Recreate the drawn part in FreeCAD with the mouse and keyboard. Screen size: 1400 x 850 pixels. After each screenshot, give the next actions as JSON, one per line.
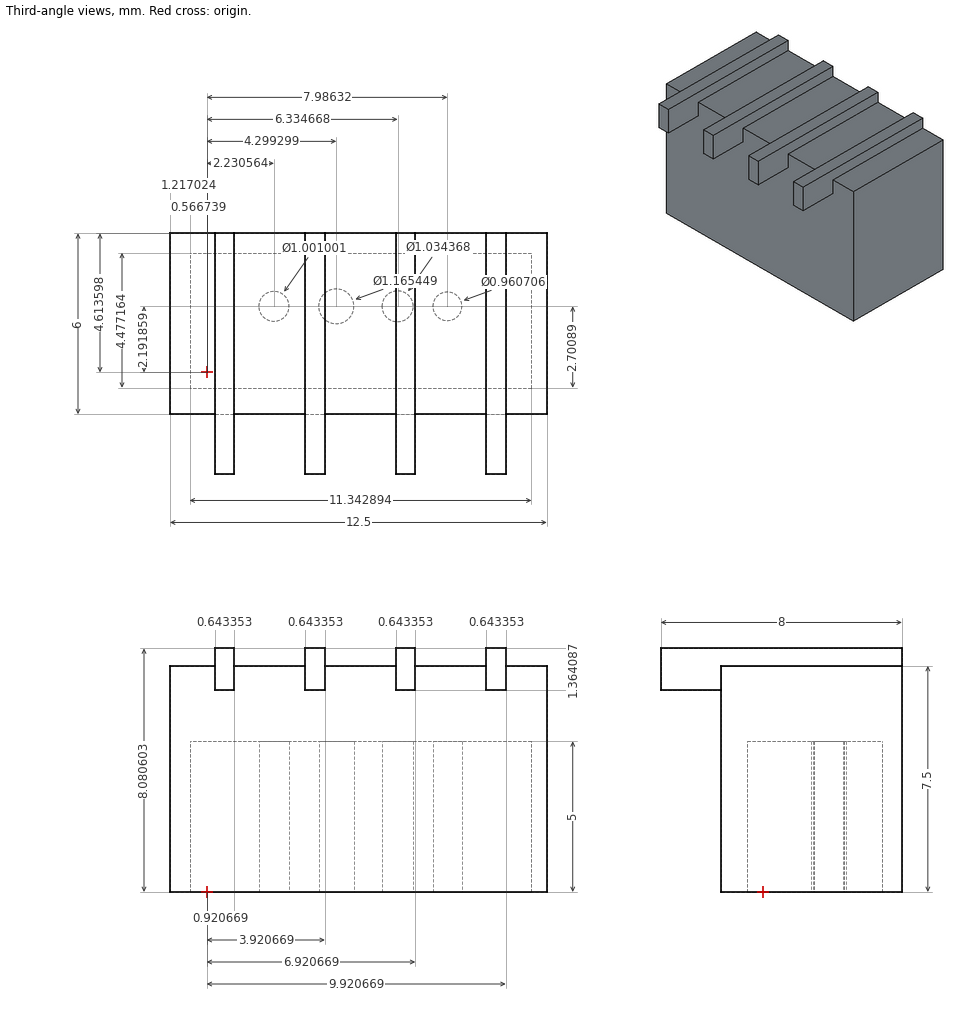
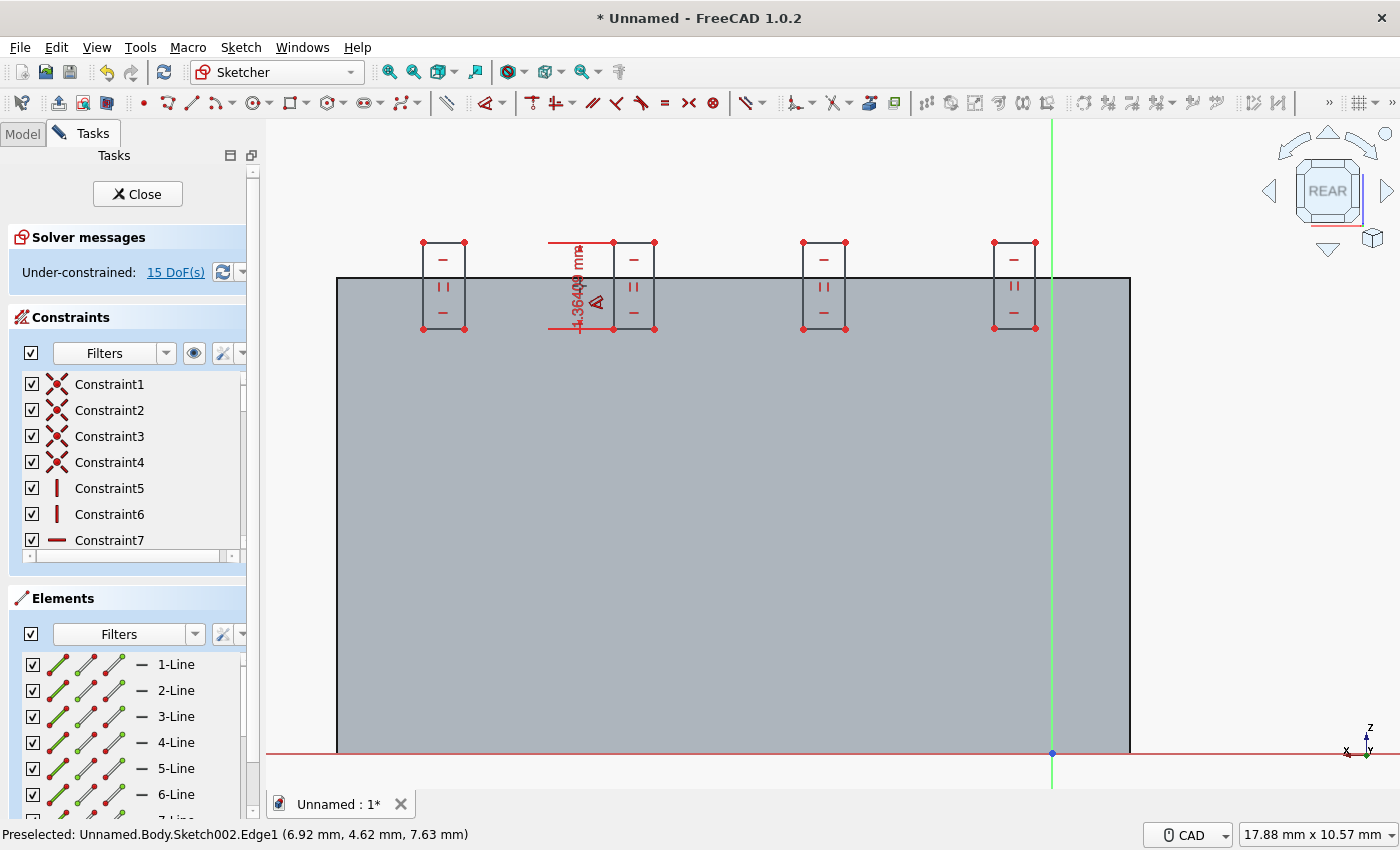
{"action": "left_click", "coordinate": [626, 329]}
{"action": "left_click", "coordinate": [634, 363]}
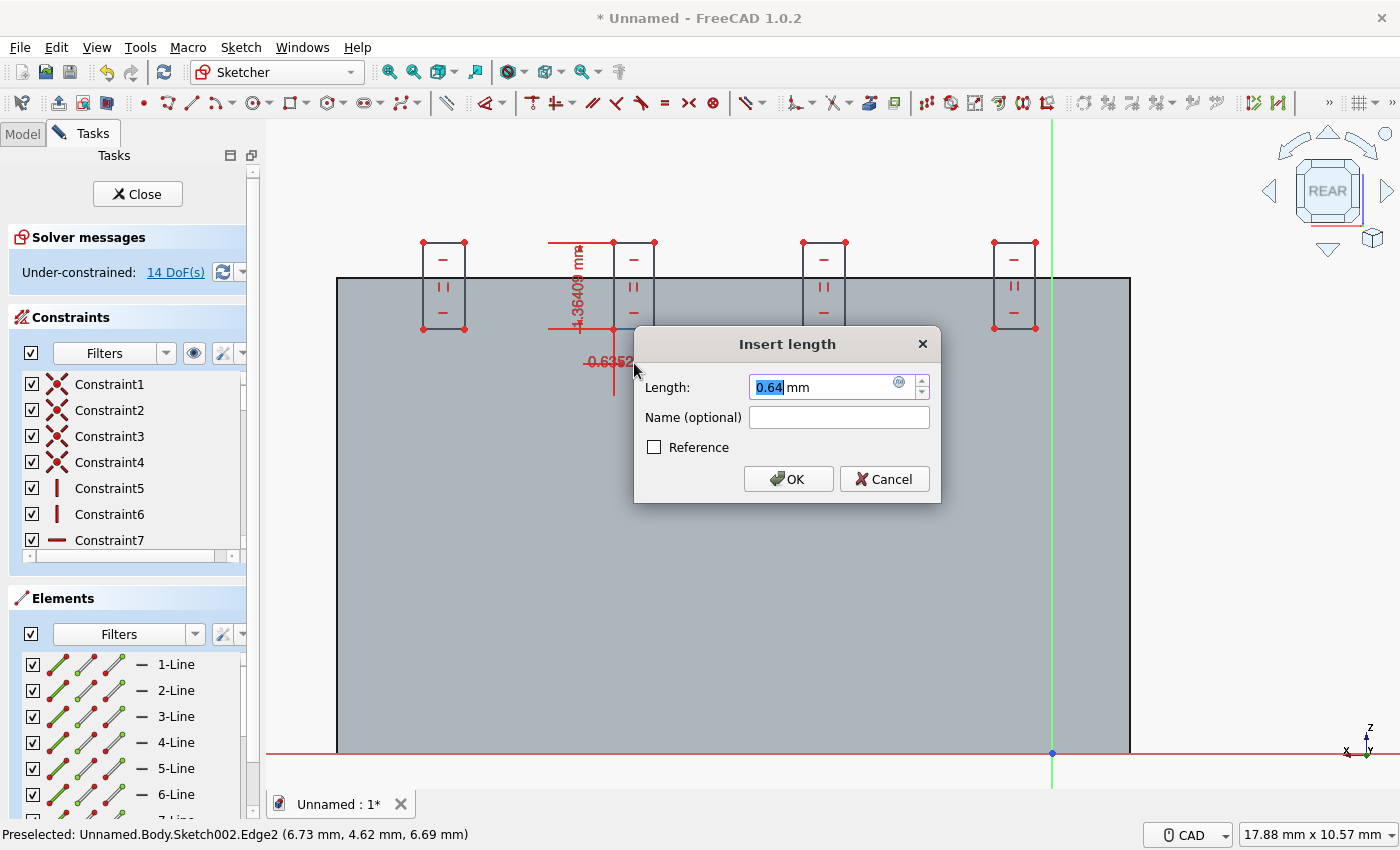
{"action": "type", "text": "0.643353"}
{"action": "key", "text": "Return"}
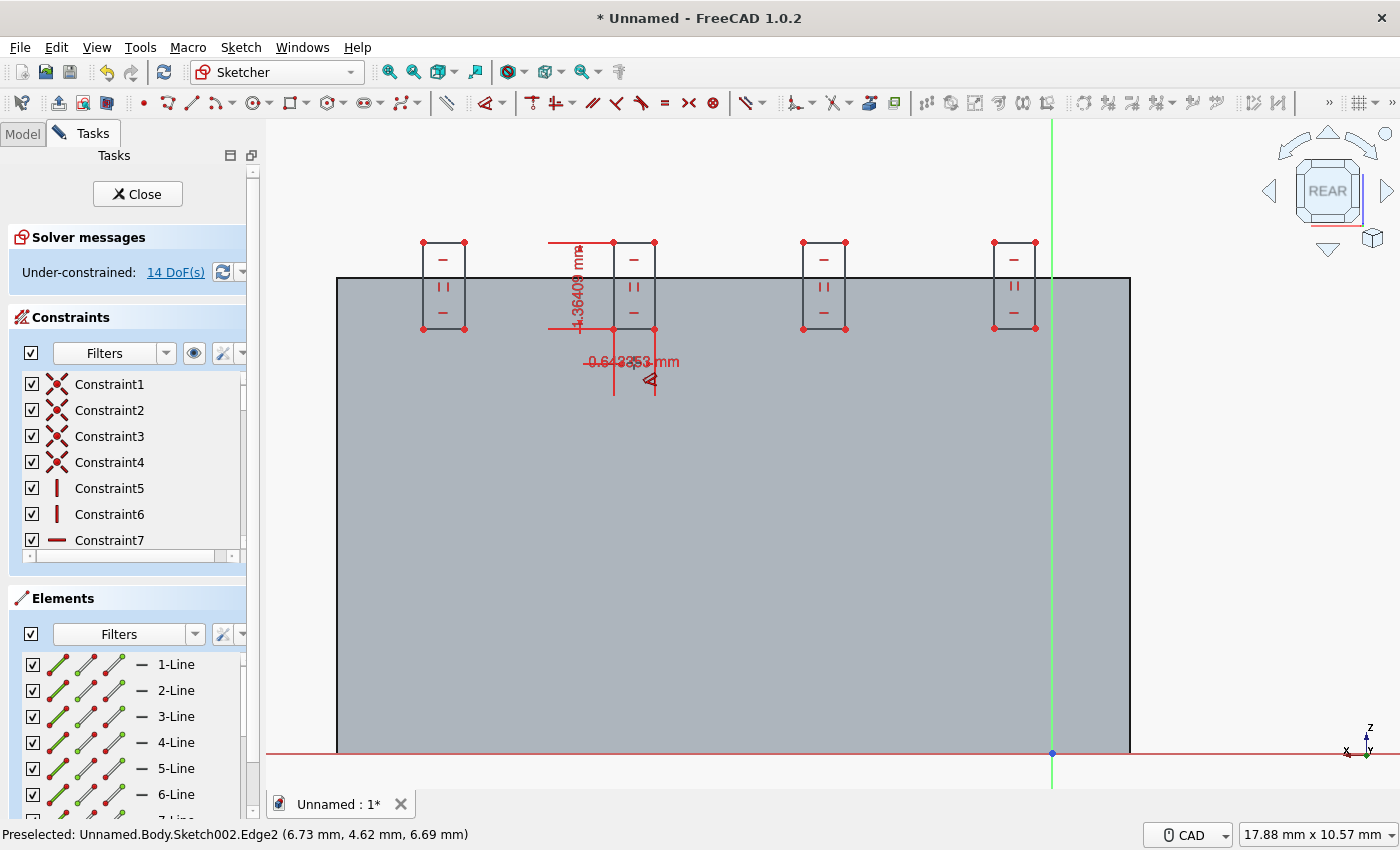
{"action": "left_click", "coordinate": [423, 269]}
{"action": "left_click", "coordinate": [389, 286]}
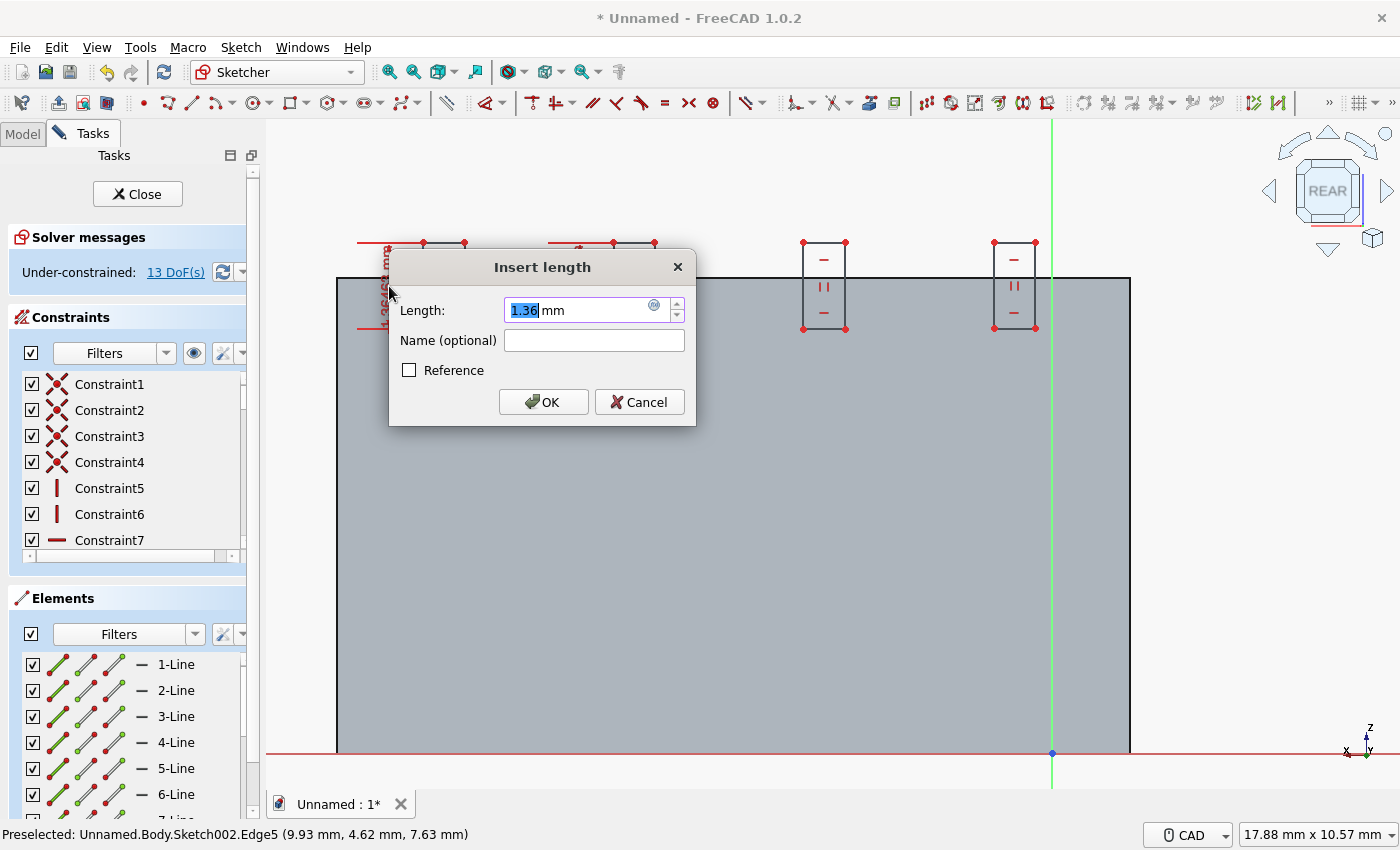
{"action": "type", "text": "1.364087"}
{"action": "key", "text": "Return"}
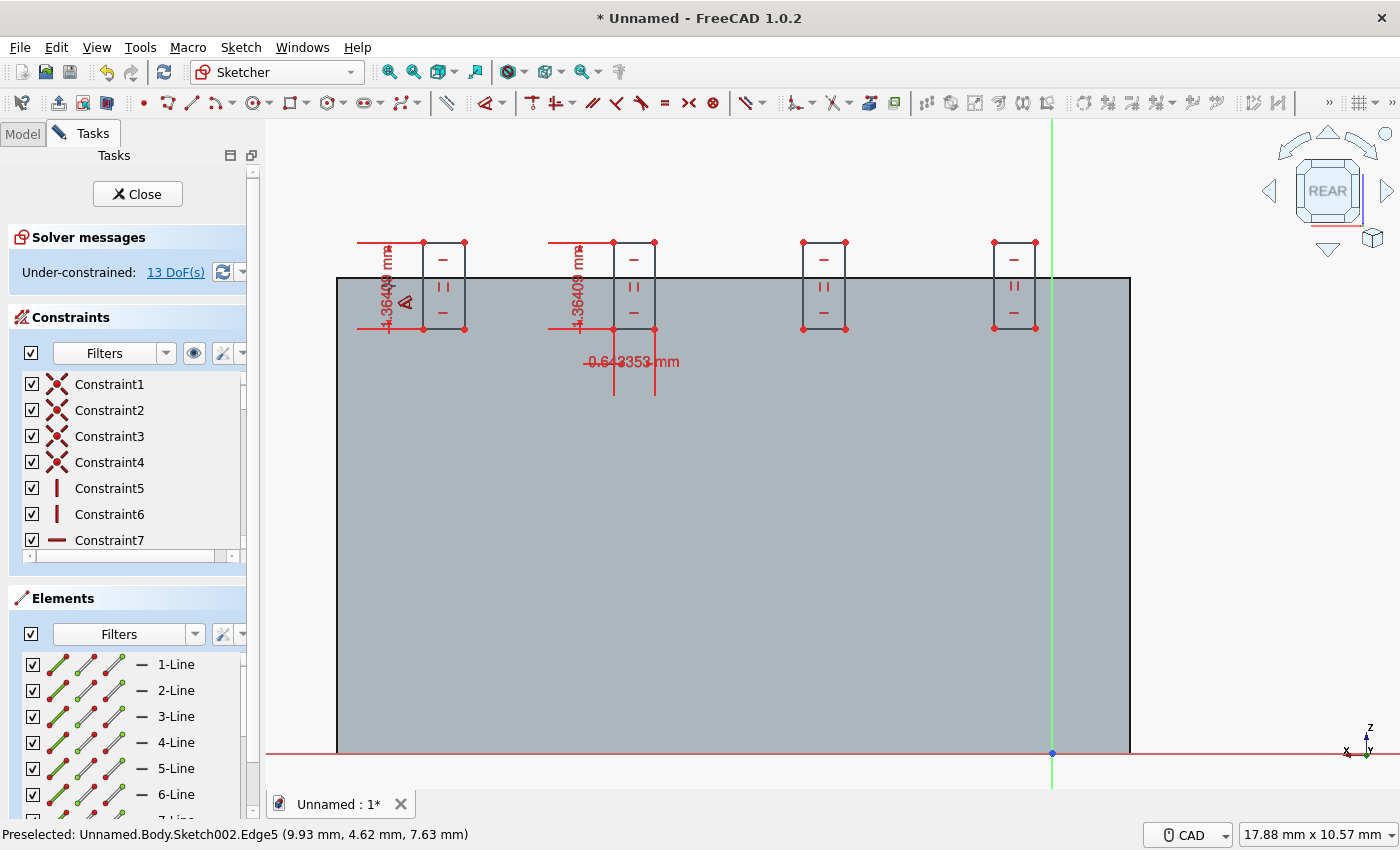
{"action": "left_click", "coordinate": [436, 329]}
{"action": "left_click", "coordinate": [444, 363]}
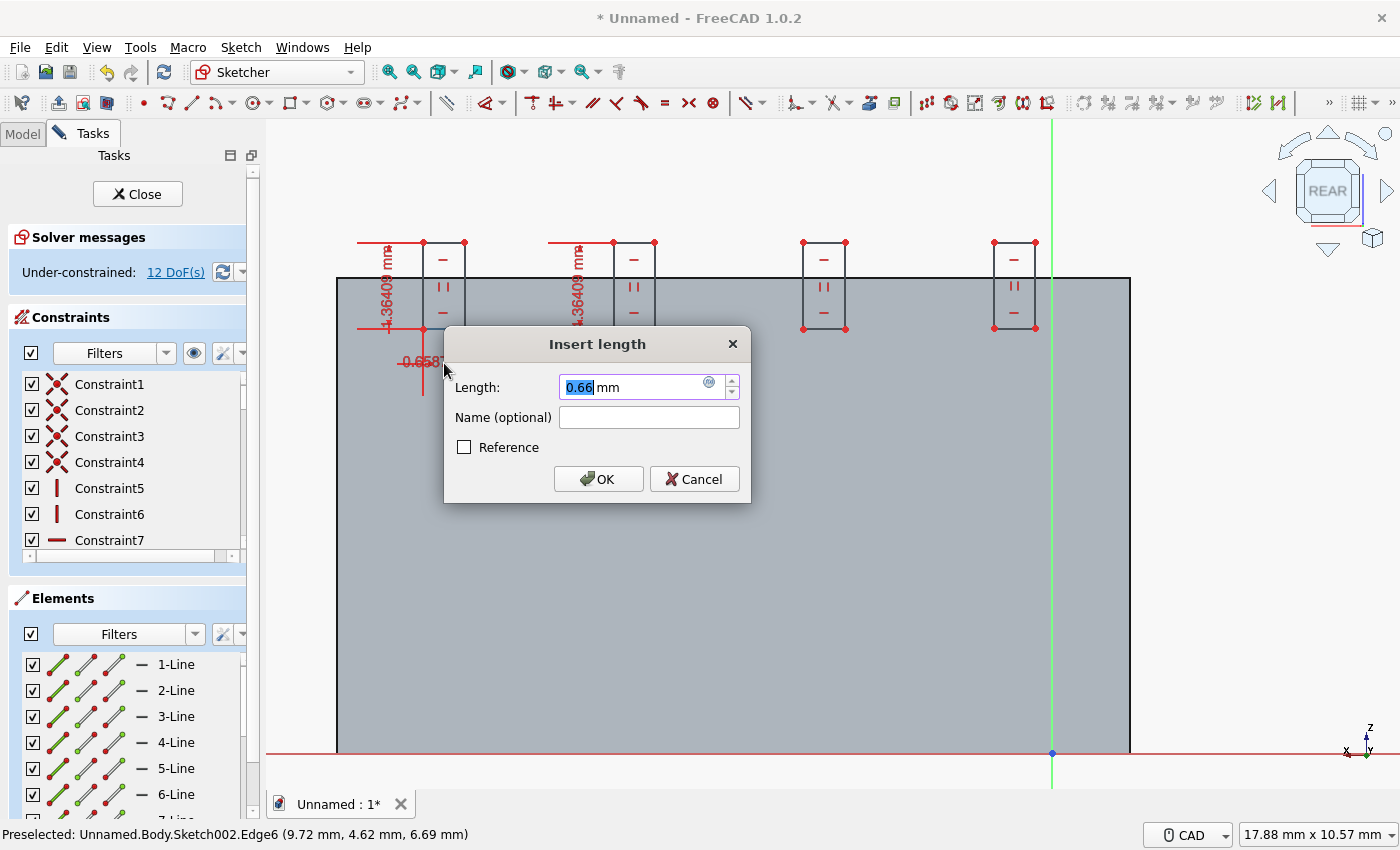
{"action": "type", "text": "0.643353"}
{"action": "key", "text": "Return"}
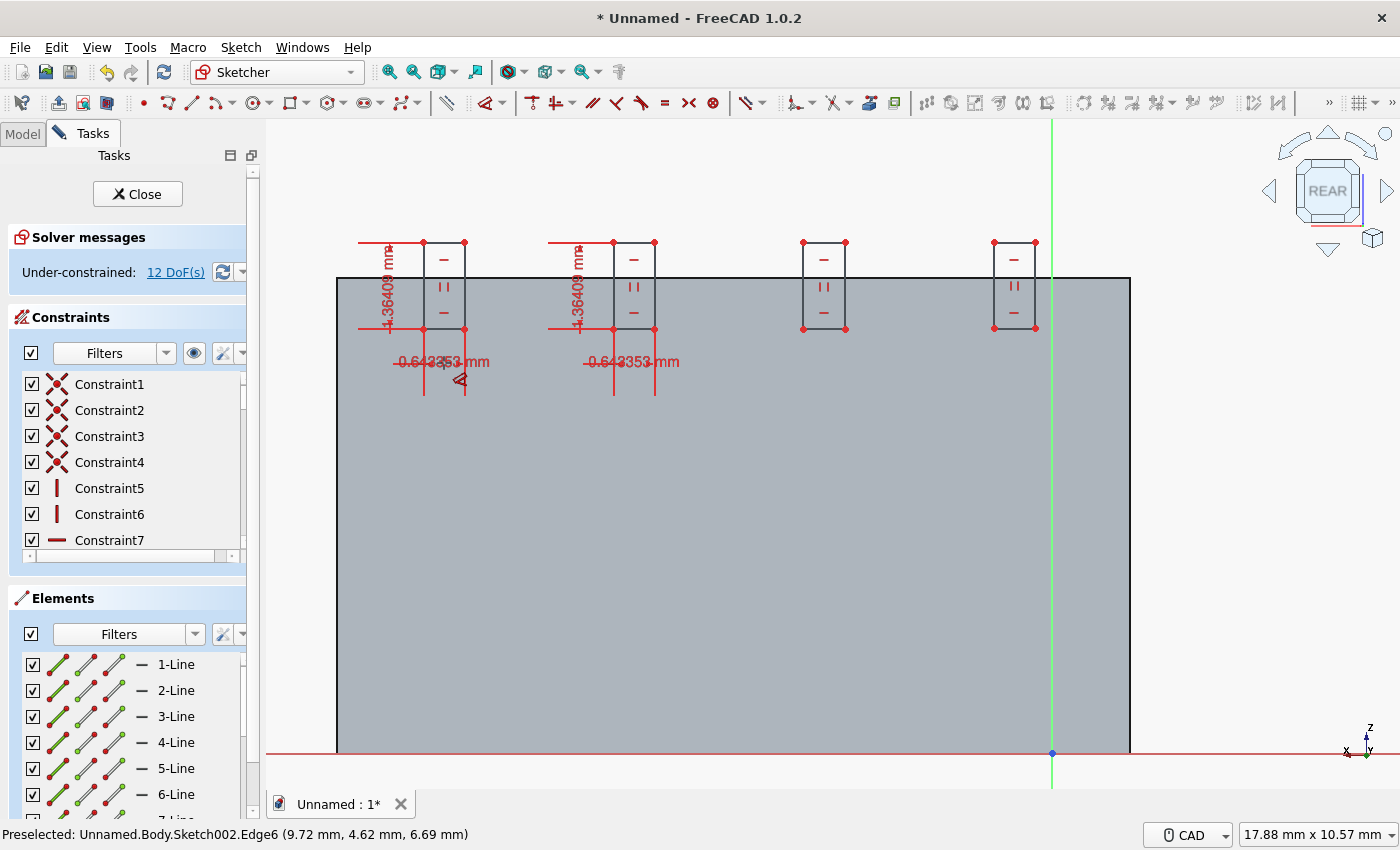
{"action": "left_click", "coordinate": [803, 269]}
{"action": "left_click", "coordinate": [769, 286]}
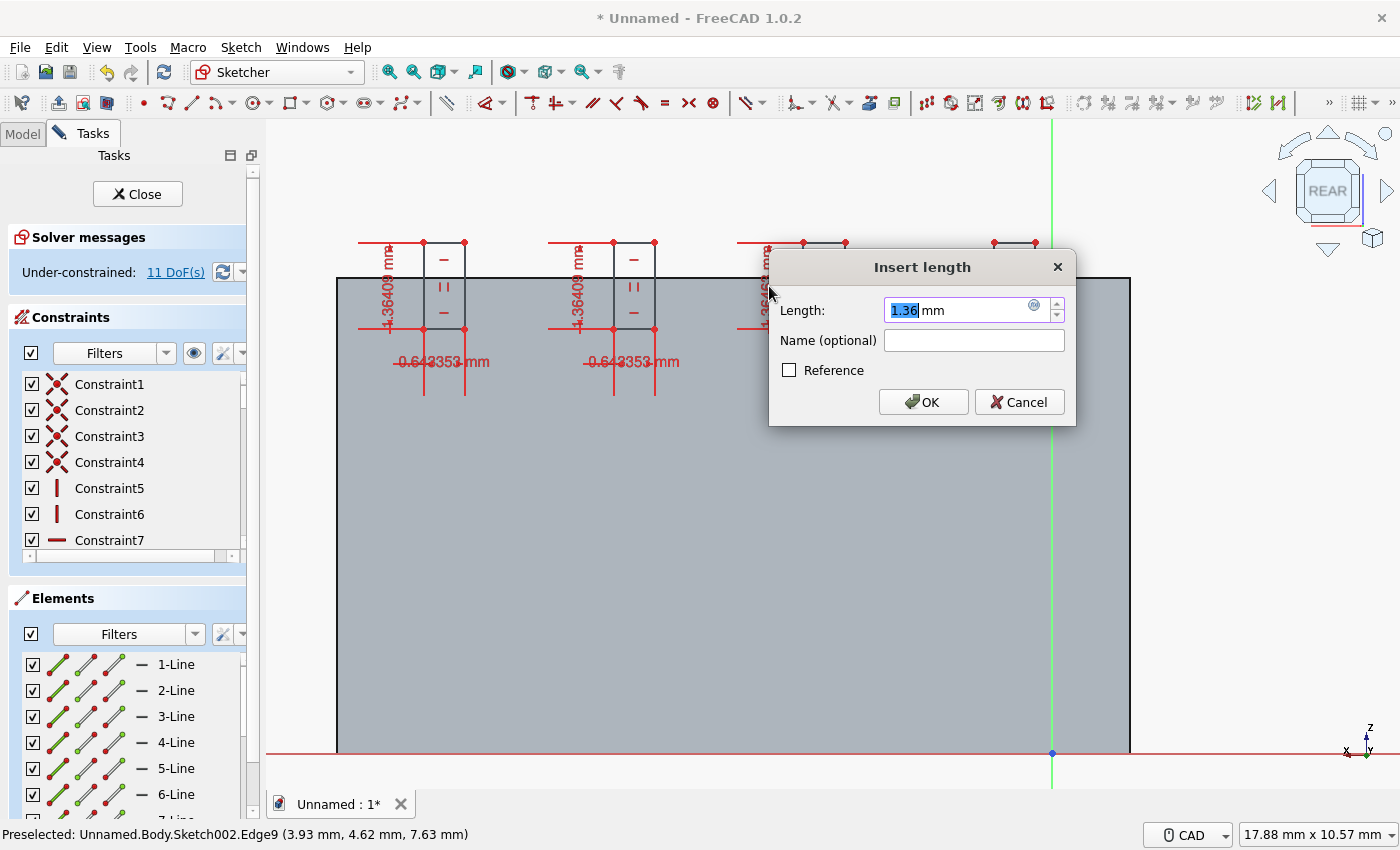
{"action": "type", "text": "1.364087"}
{"action": "key", "text": "Return"}